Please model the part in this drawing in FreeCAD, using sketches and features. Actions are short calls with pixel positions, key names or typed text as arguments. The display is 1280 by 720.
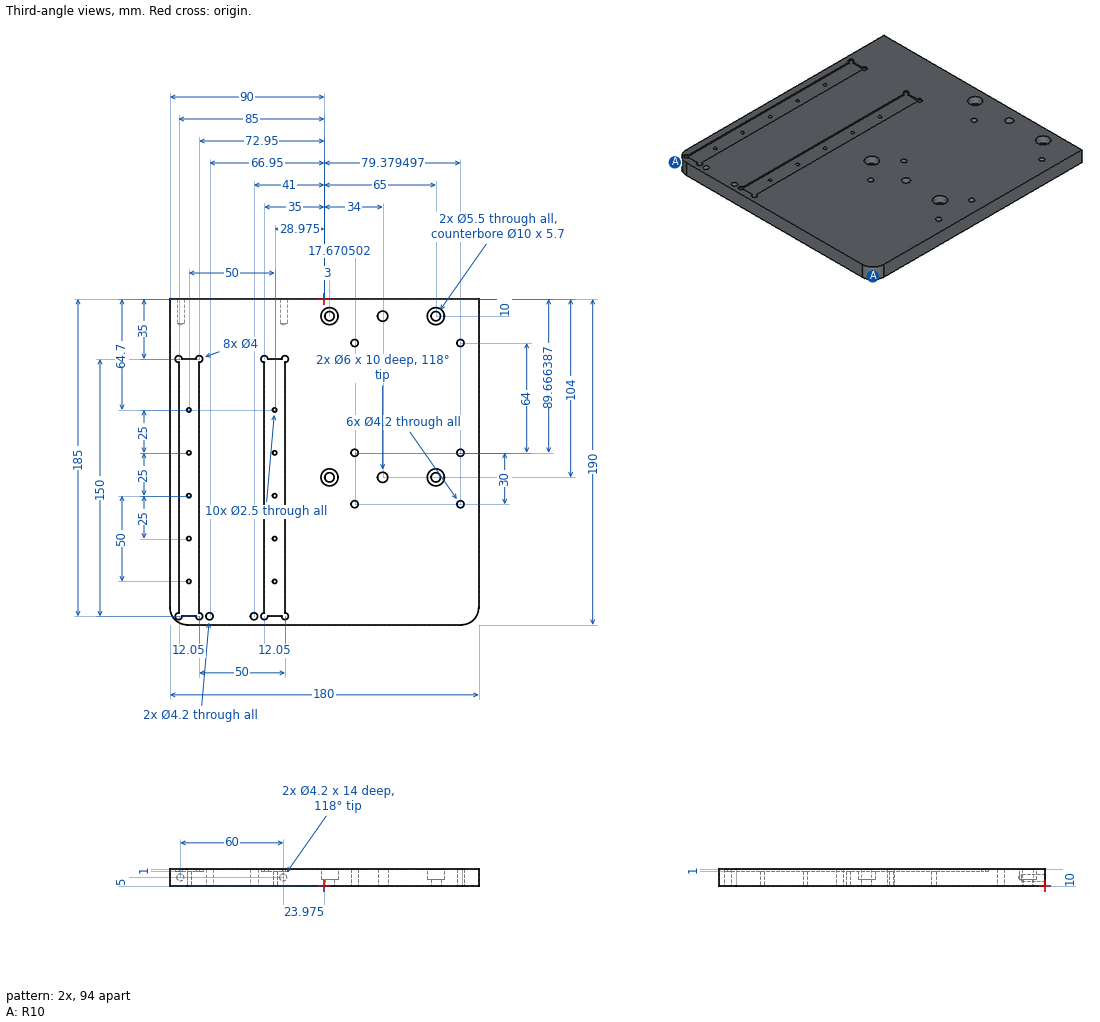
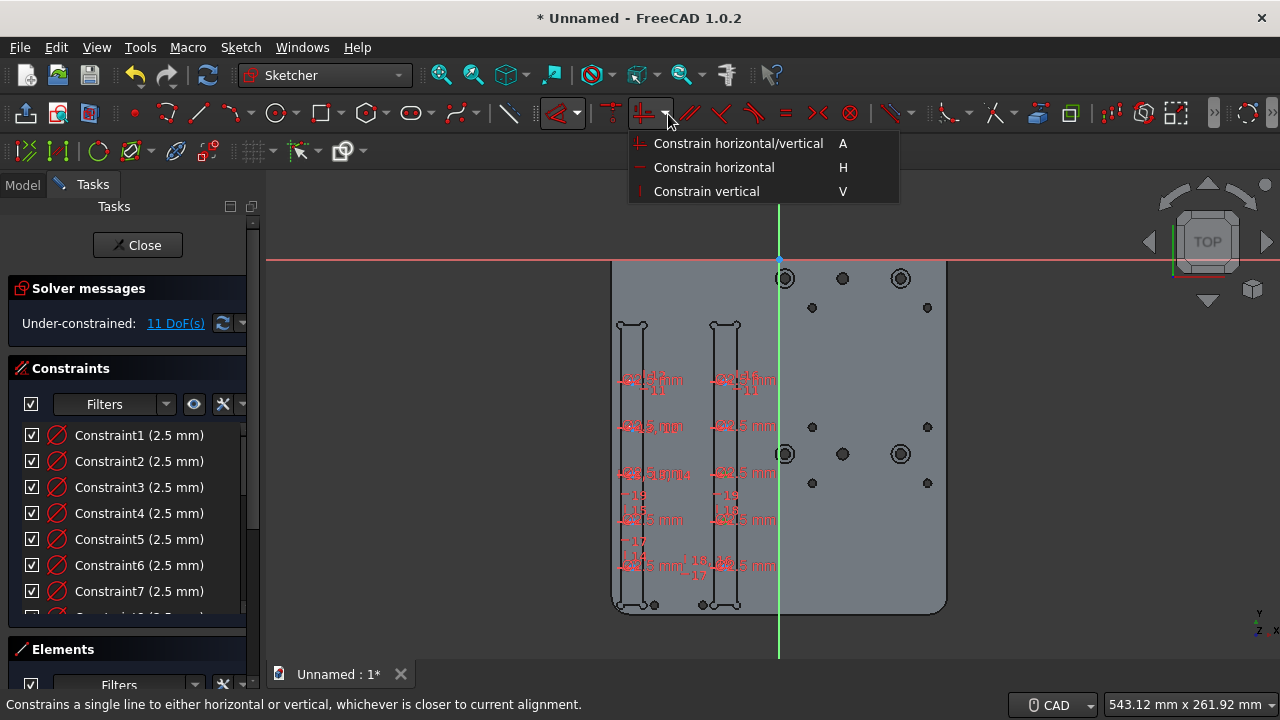
click(764, 191)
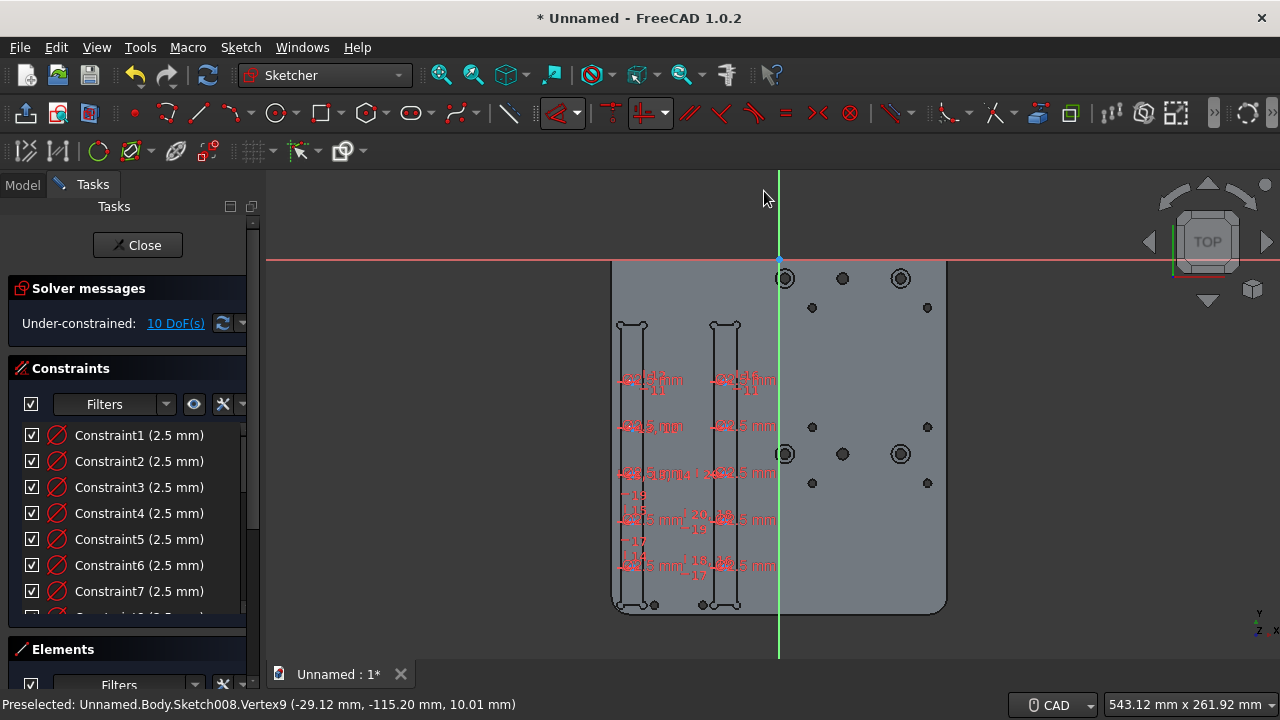
click(632, 475)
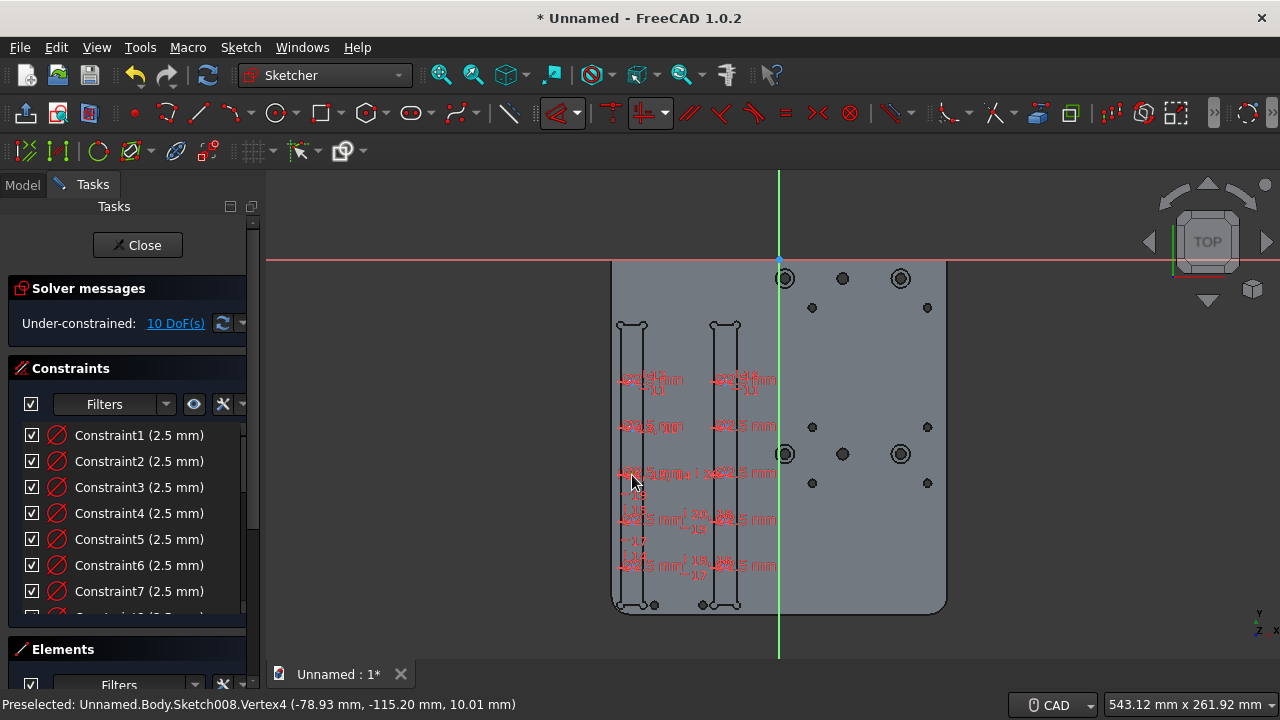
click(725, 475)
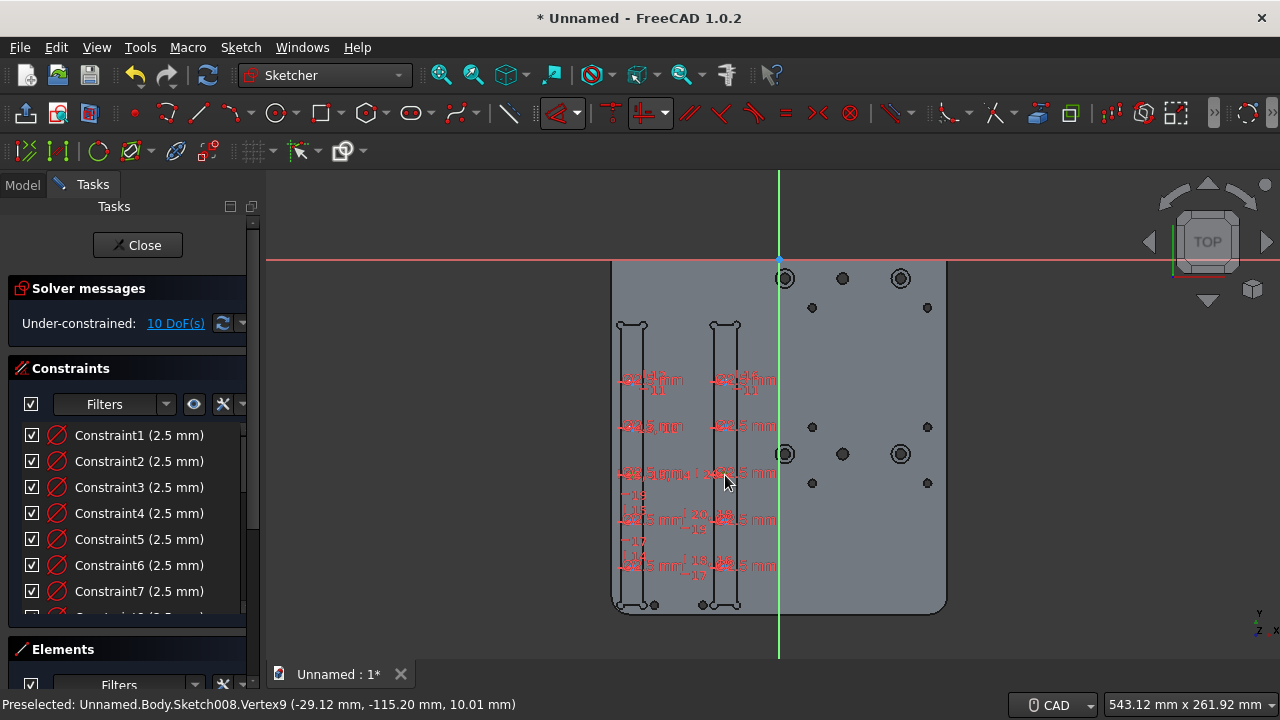
key(h)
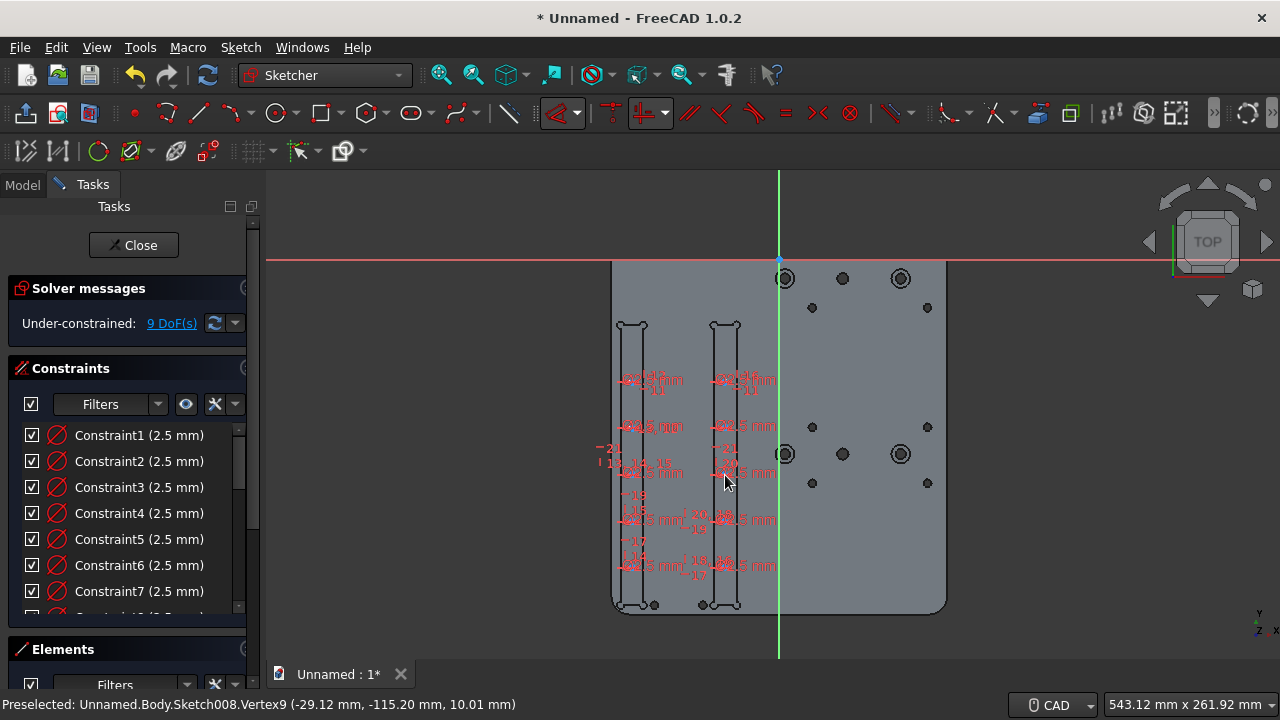
click(725, 382)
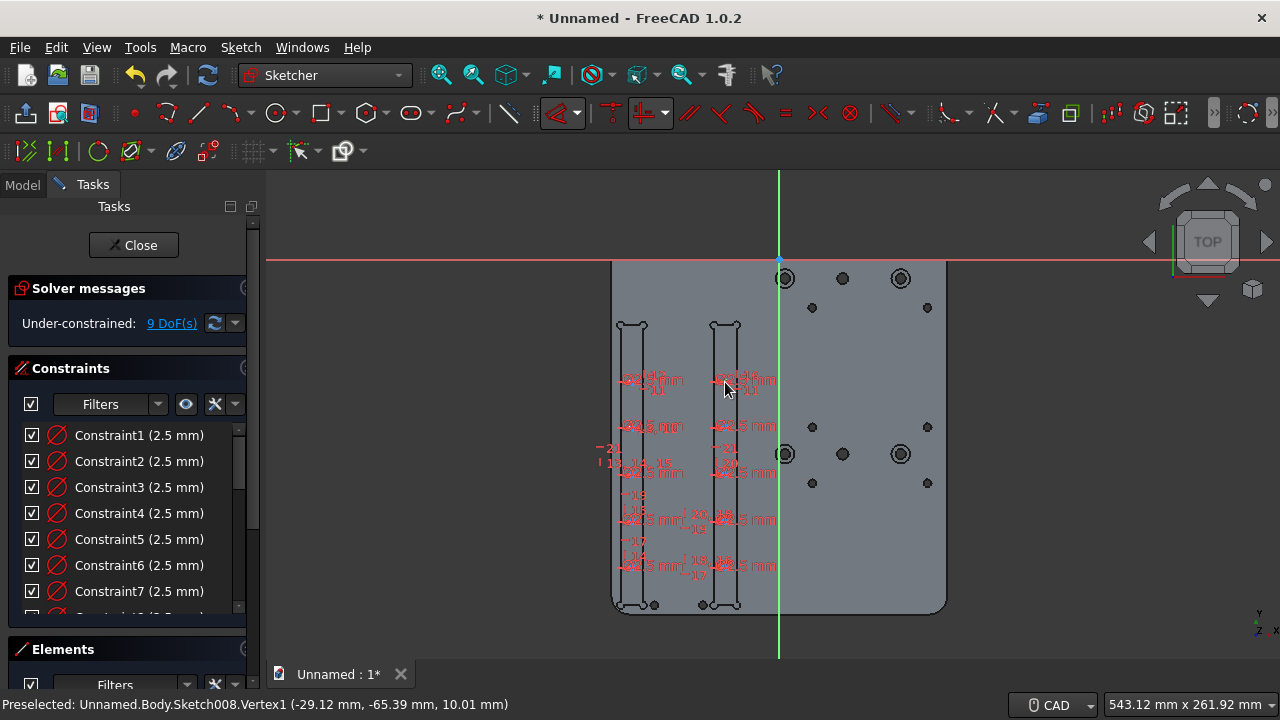
click(725, 428)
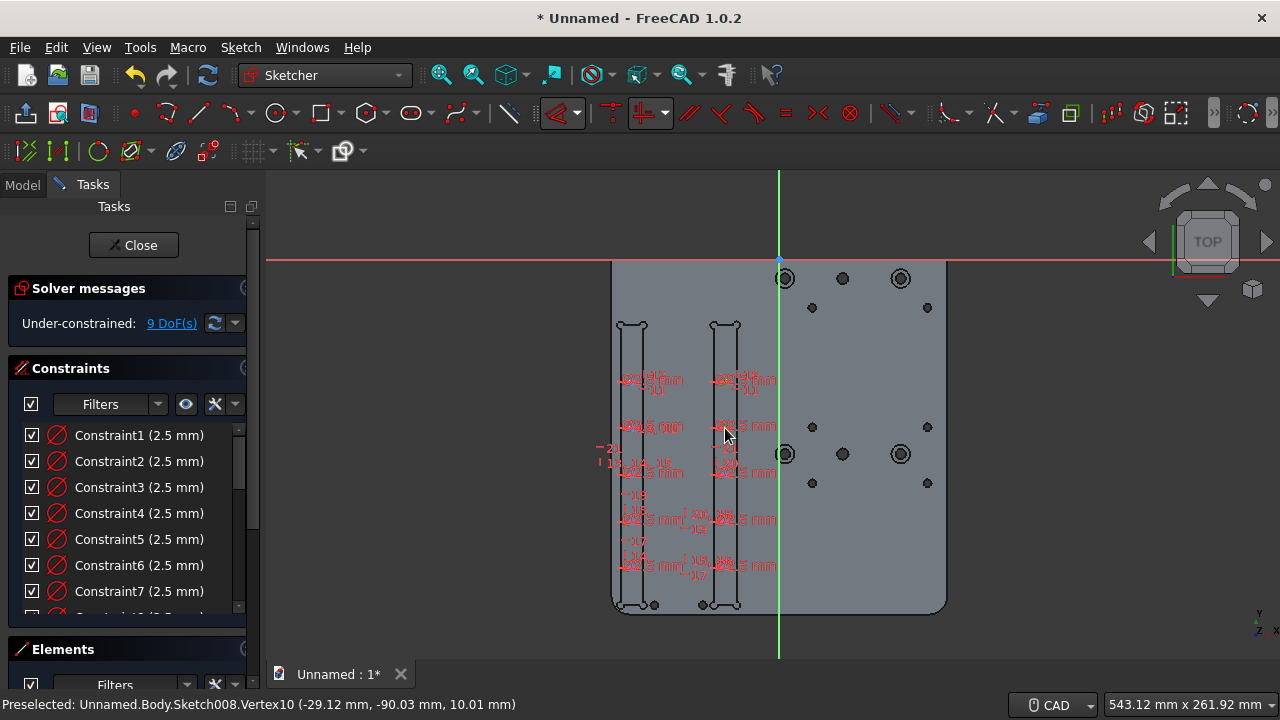
key(v)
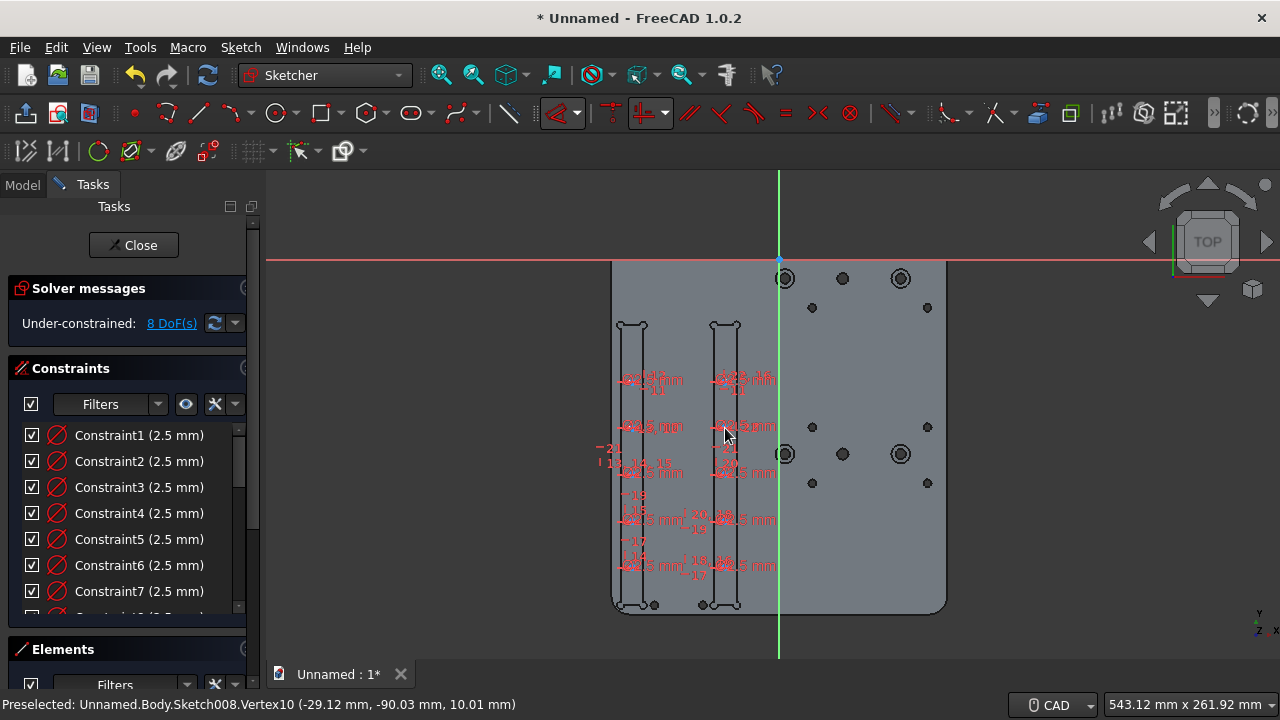
click(632, 428)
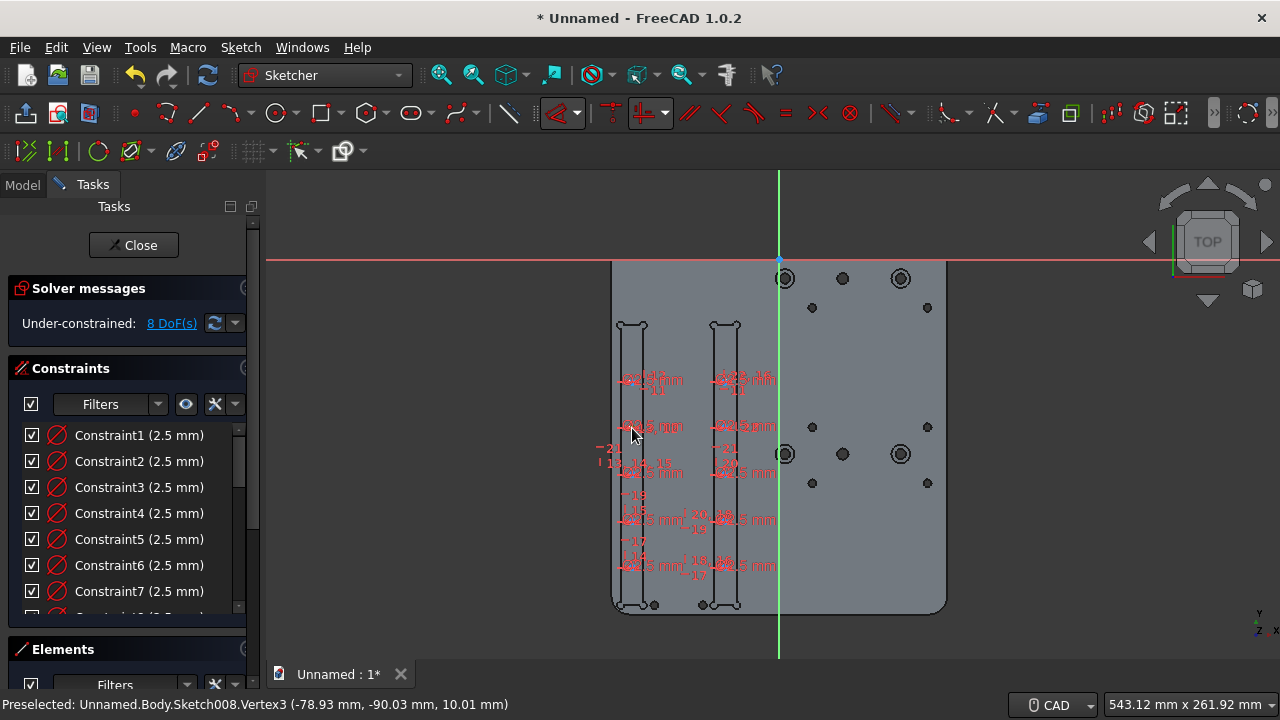
click(725, 428)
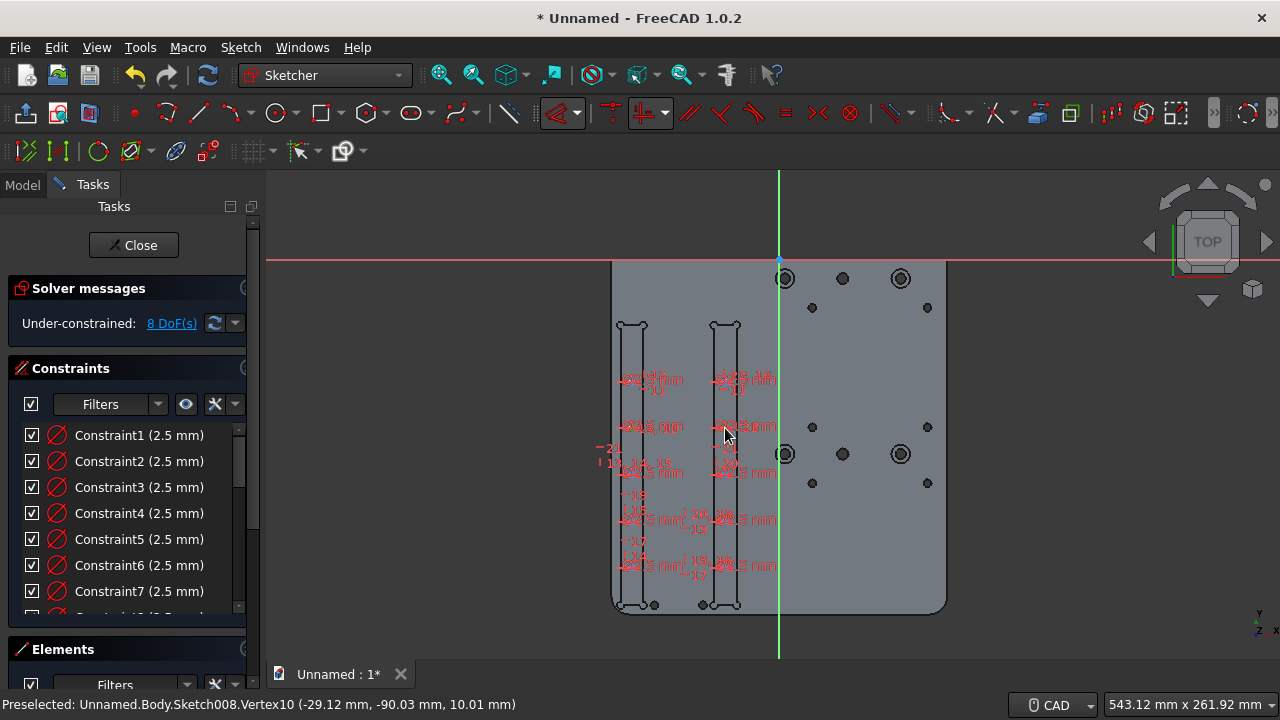
key(h)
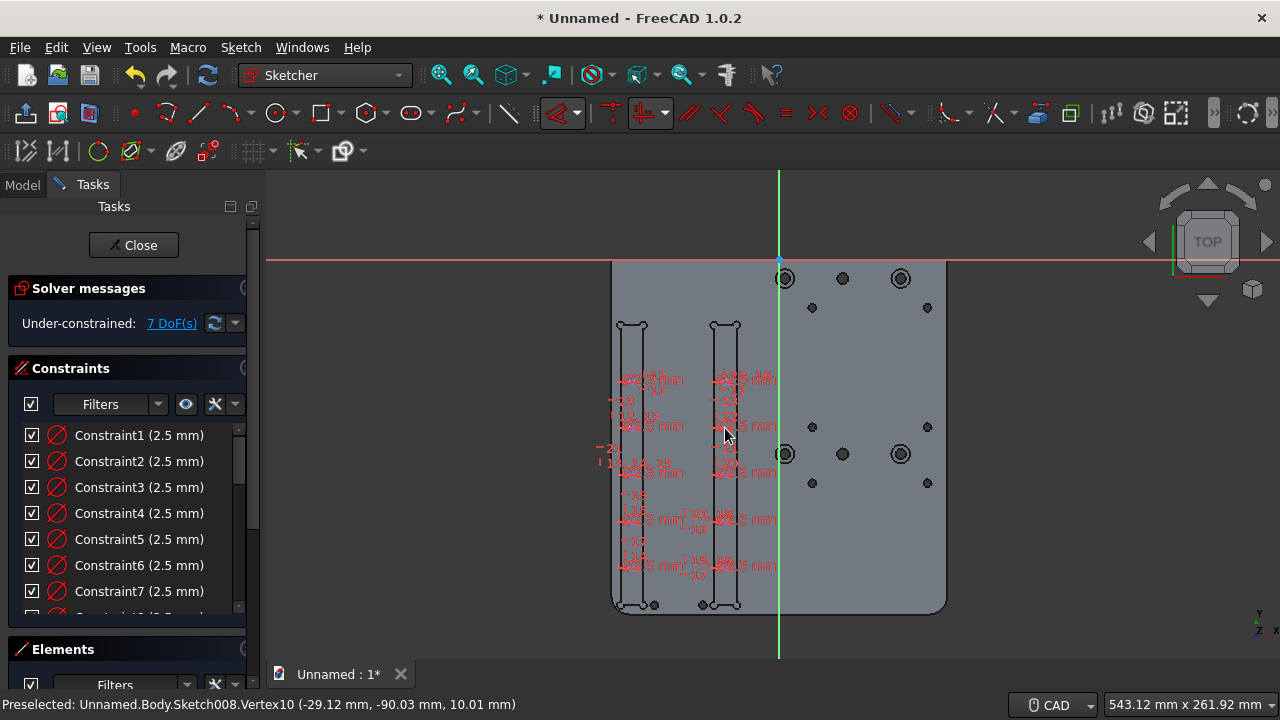
click(725, 382)